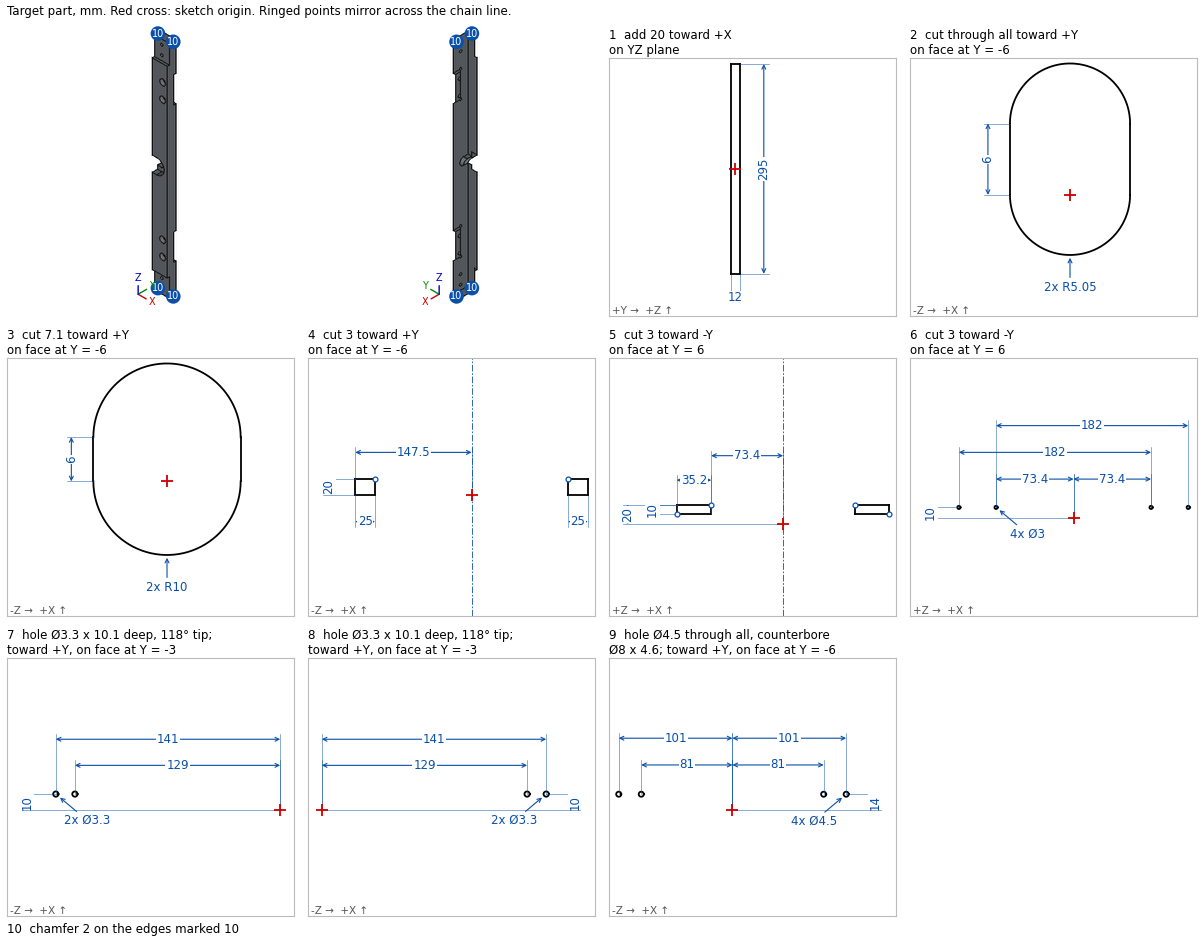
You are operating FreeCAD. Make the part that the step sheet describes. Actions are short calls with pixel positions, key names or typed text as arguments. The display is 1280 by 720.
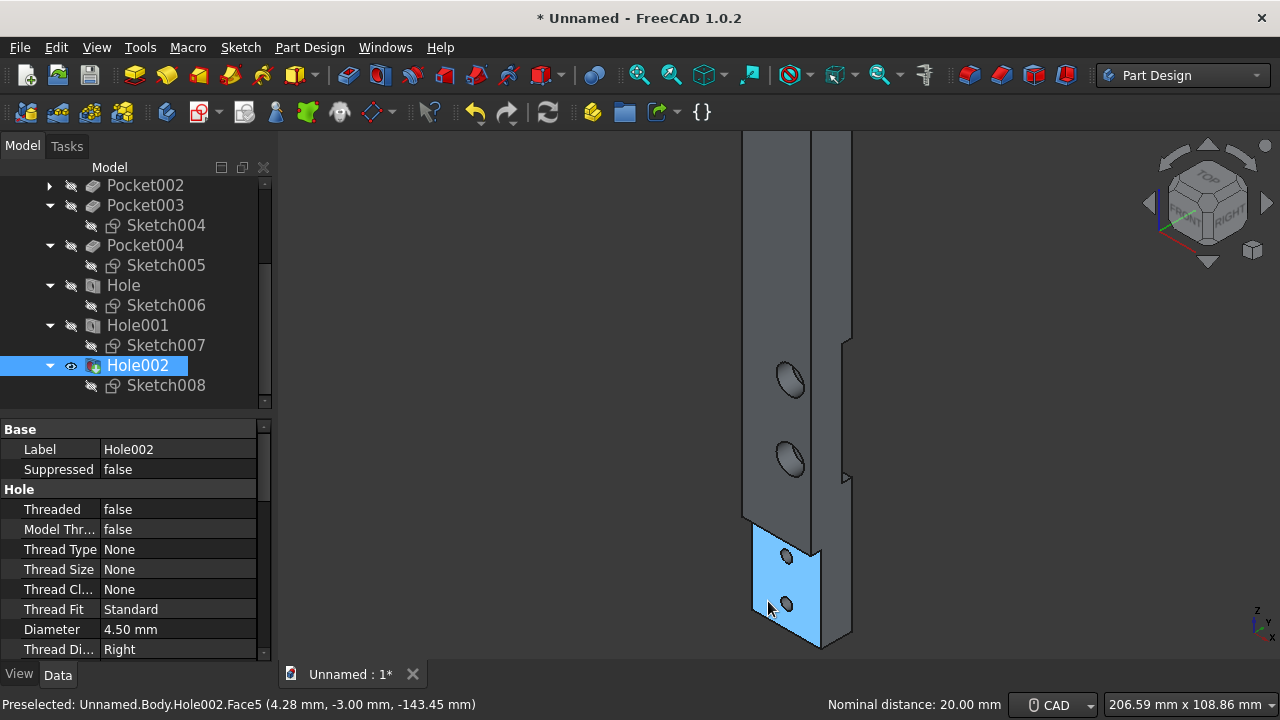
click(640, 76)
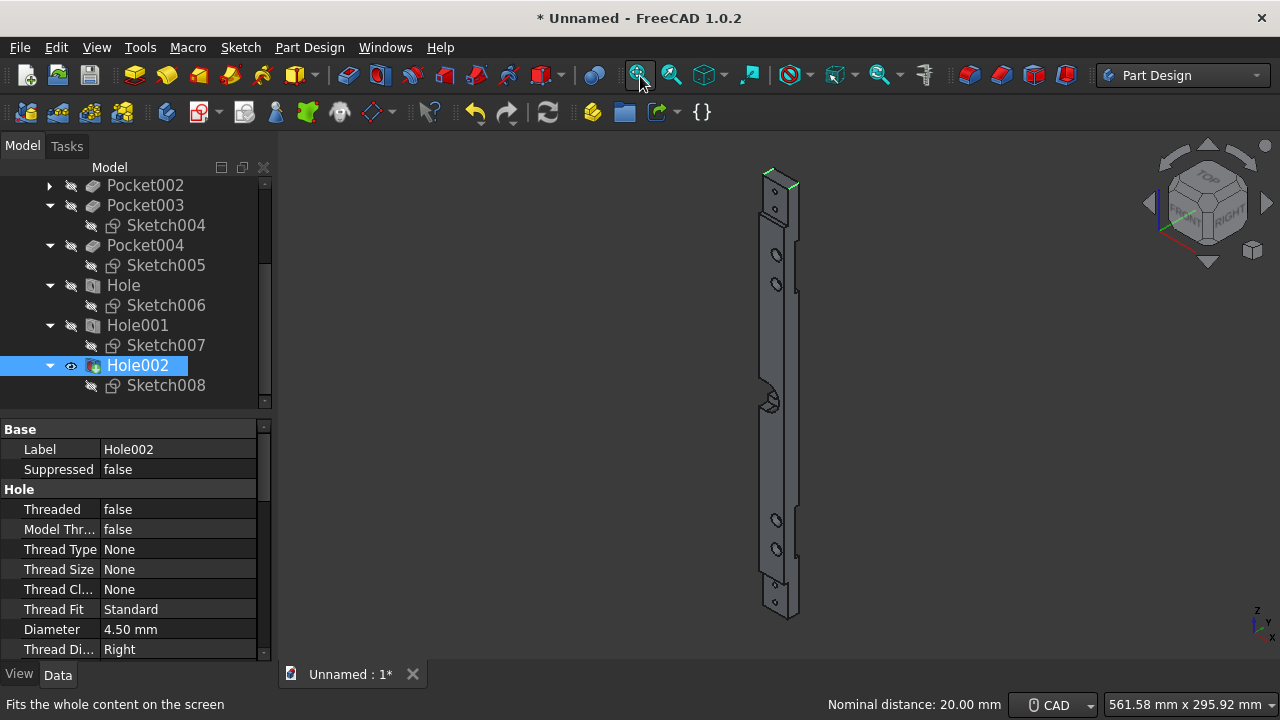
key(1)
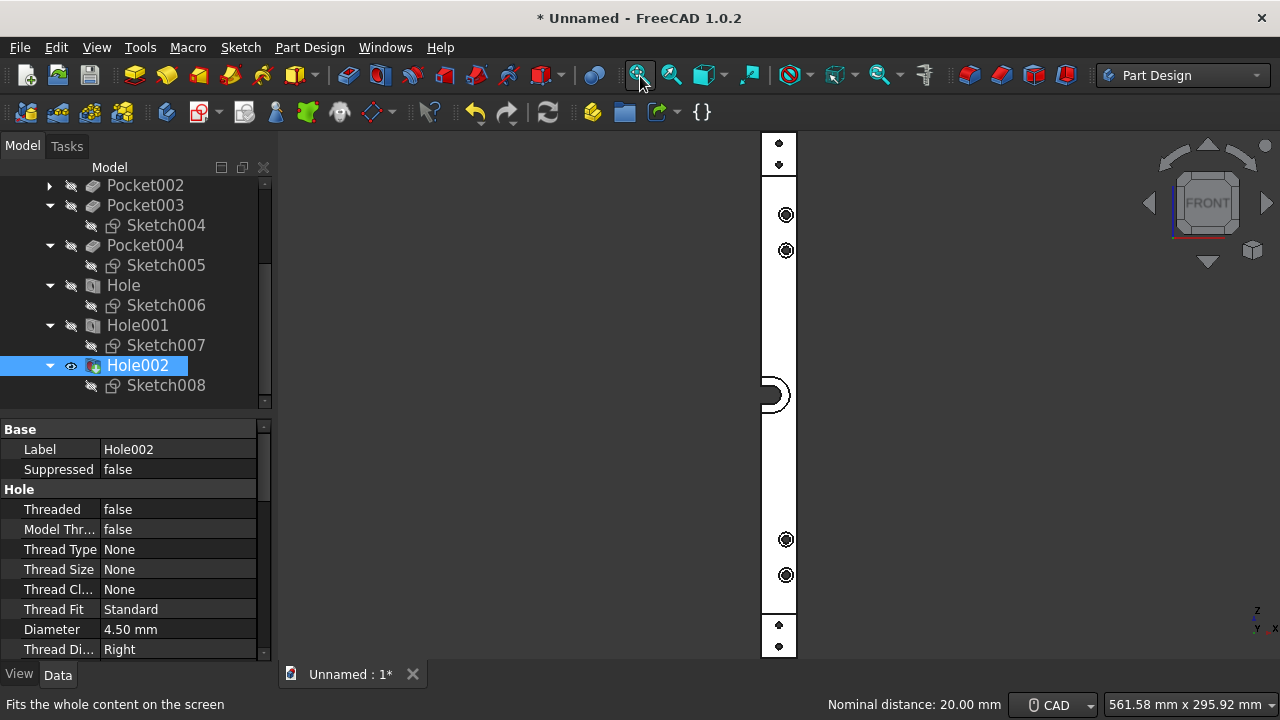
key(3)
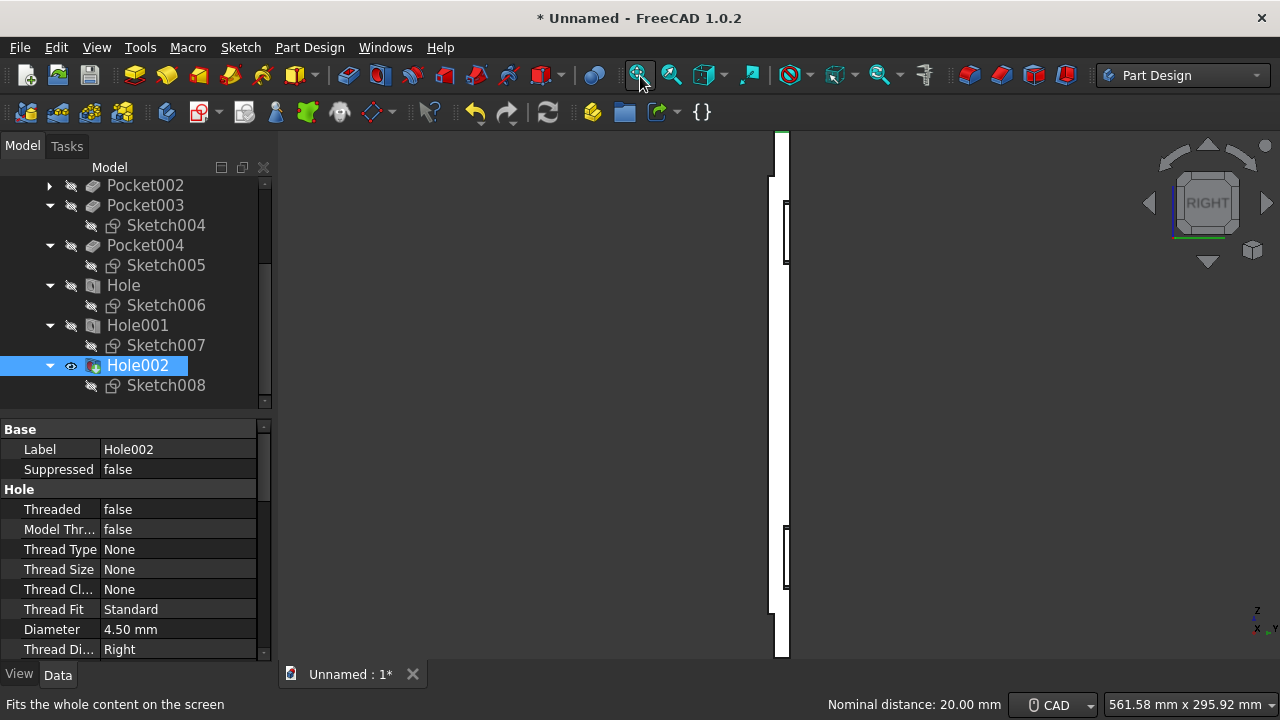
key(5)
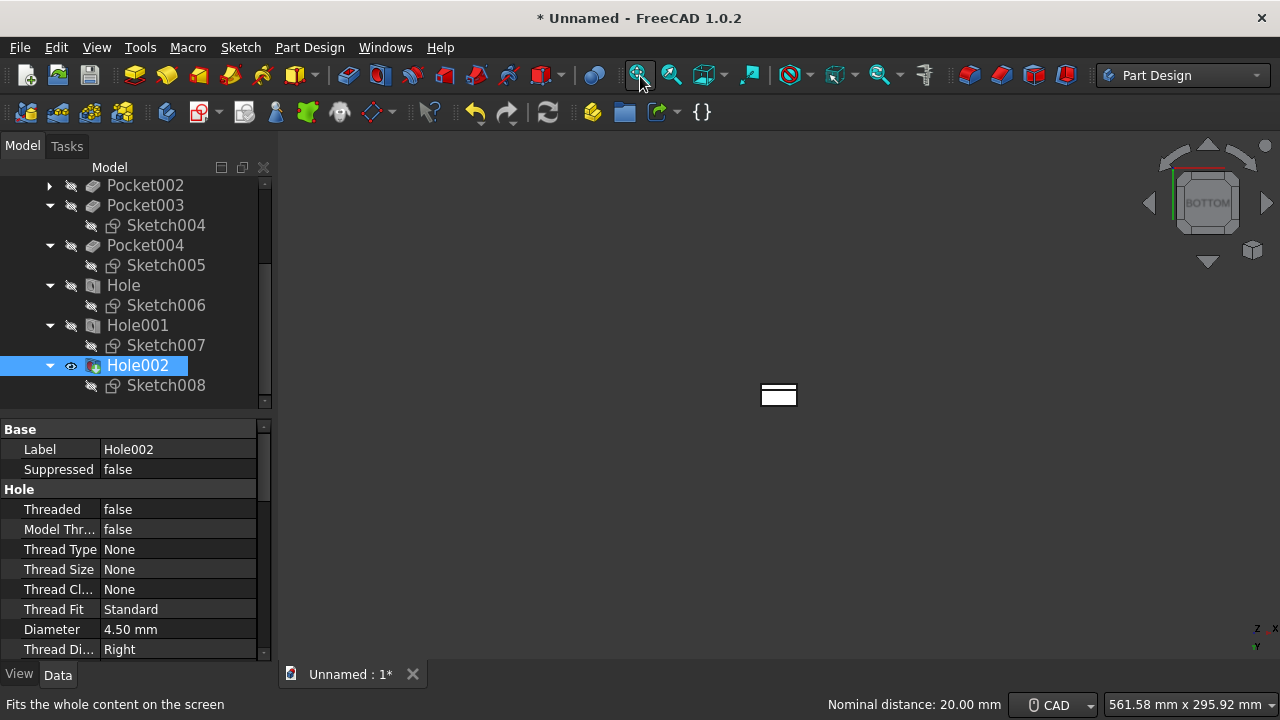
click(640, 76)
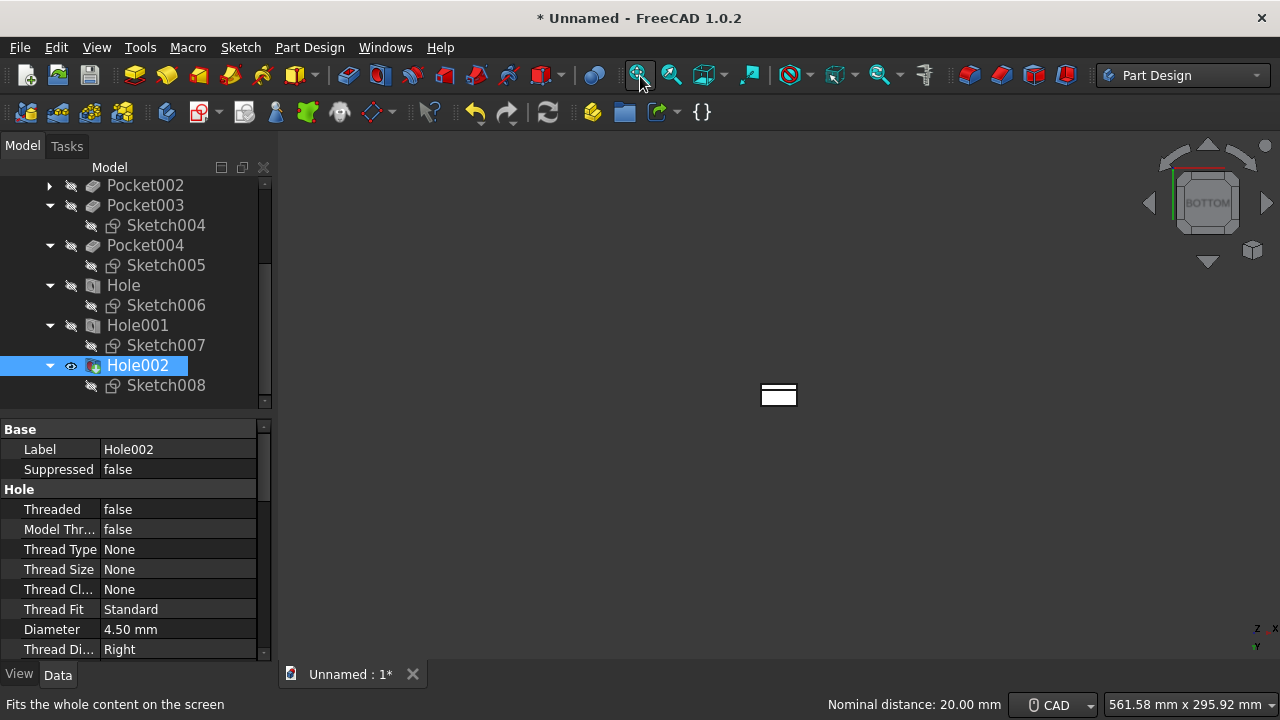
click(761, 397, ctrl)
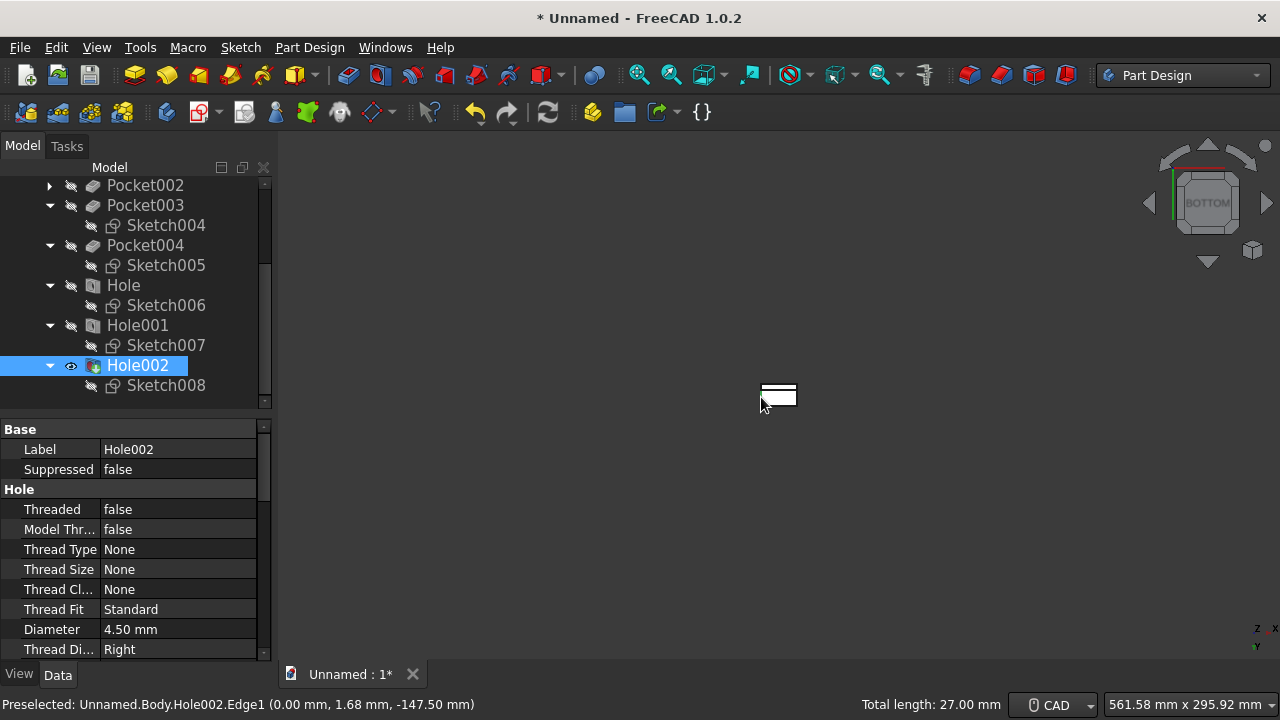
click(797, 397, ctrl)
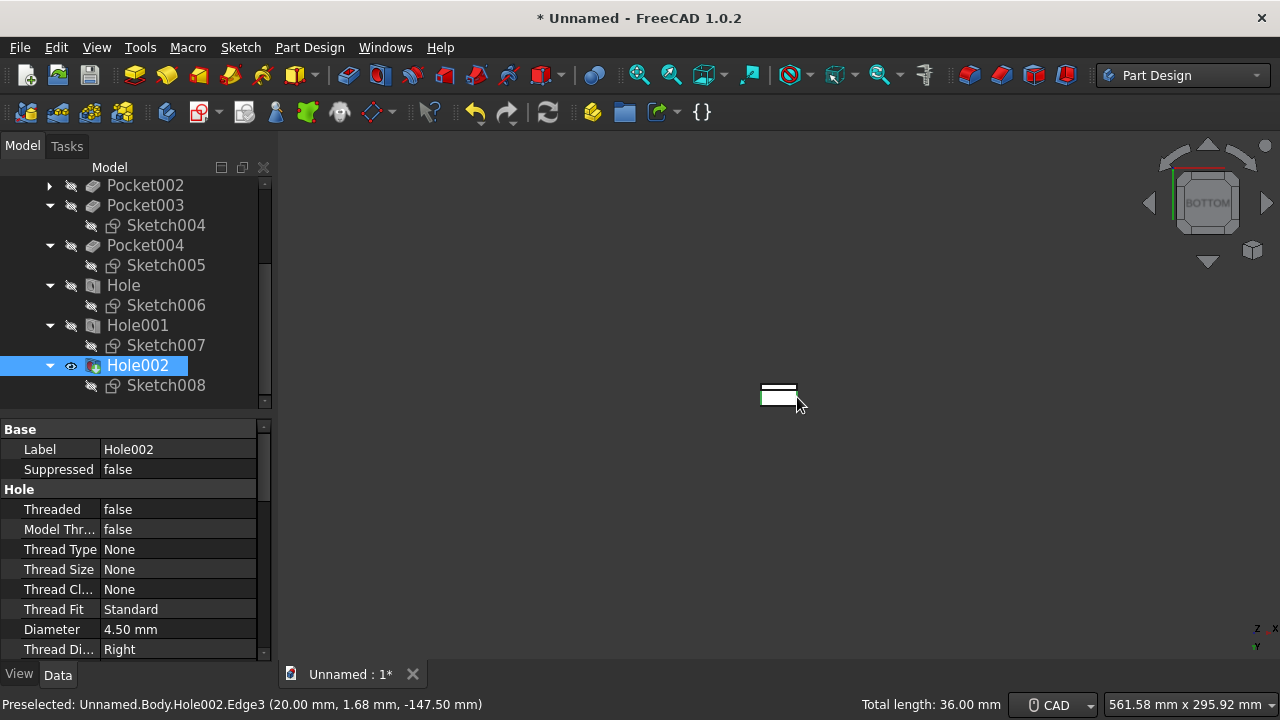
click(1002, 76)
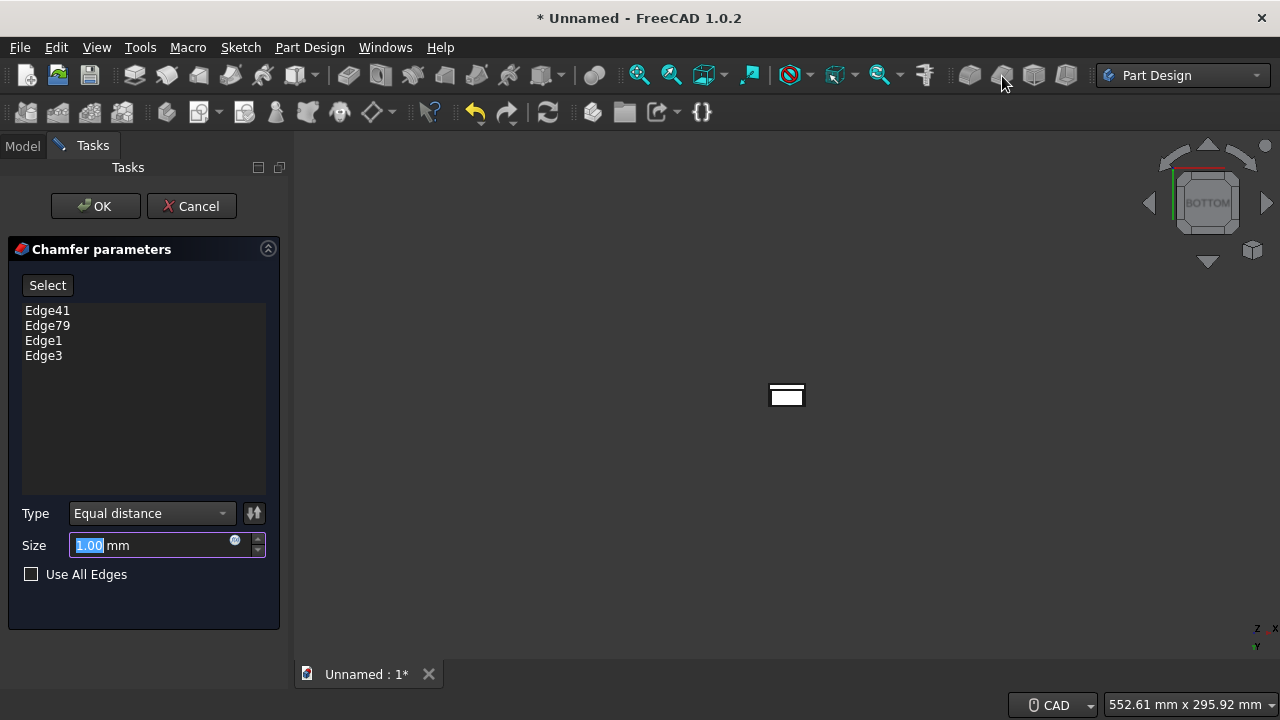
text(2)
key(Tab)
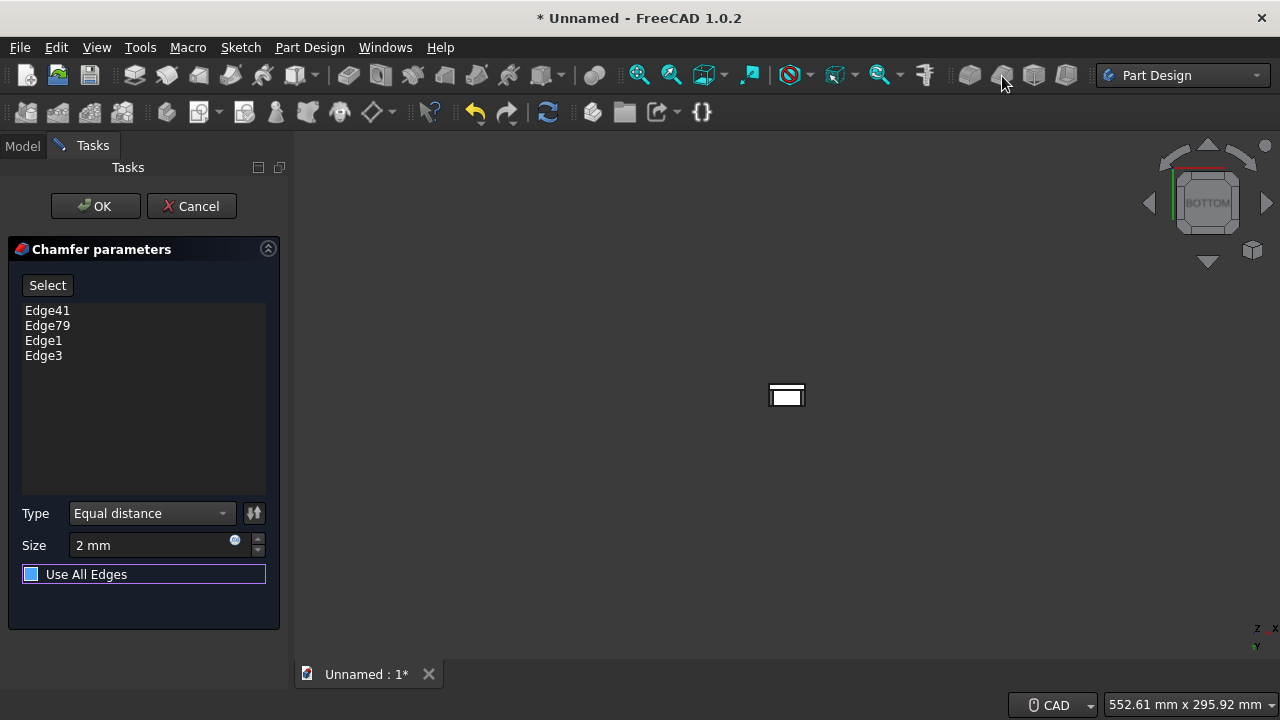
click(96, 206)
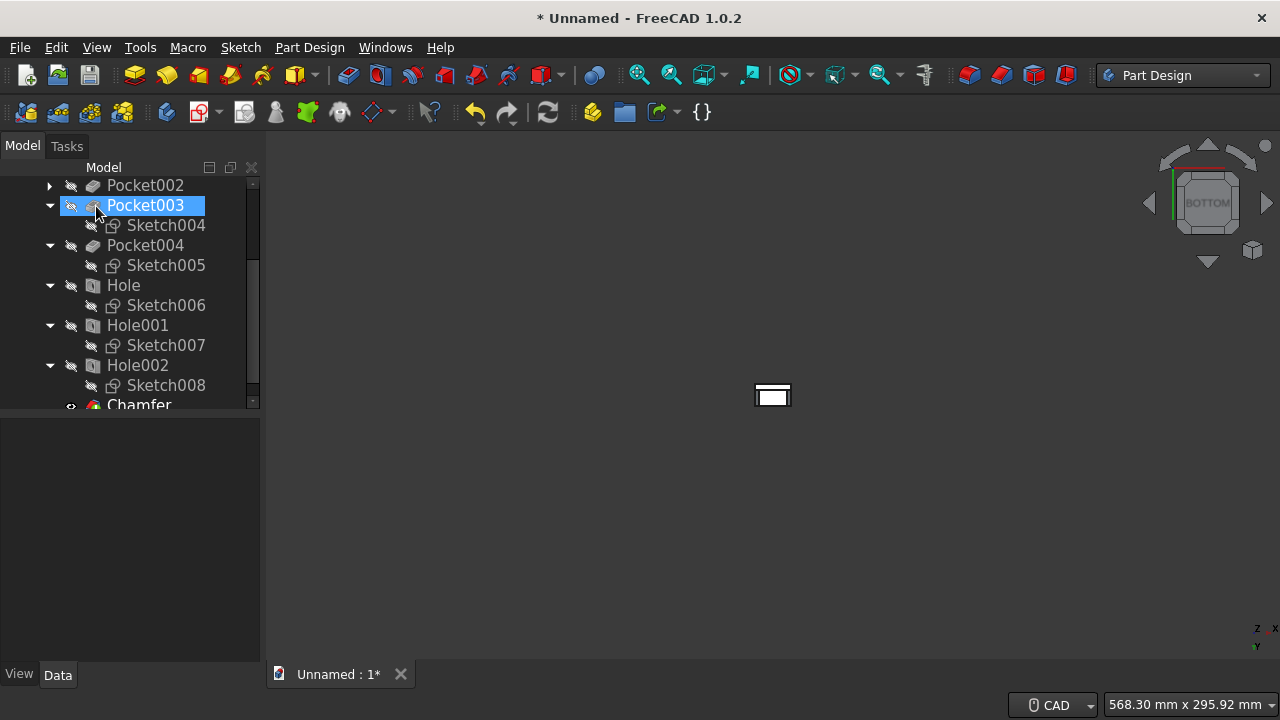
key(0)